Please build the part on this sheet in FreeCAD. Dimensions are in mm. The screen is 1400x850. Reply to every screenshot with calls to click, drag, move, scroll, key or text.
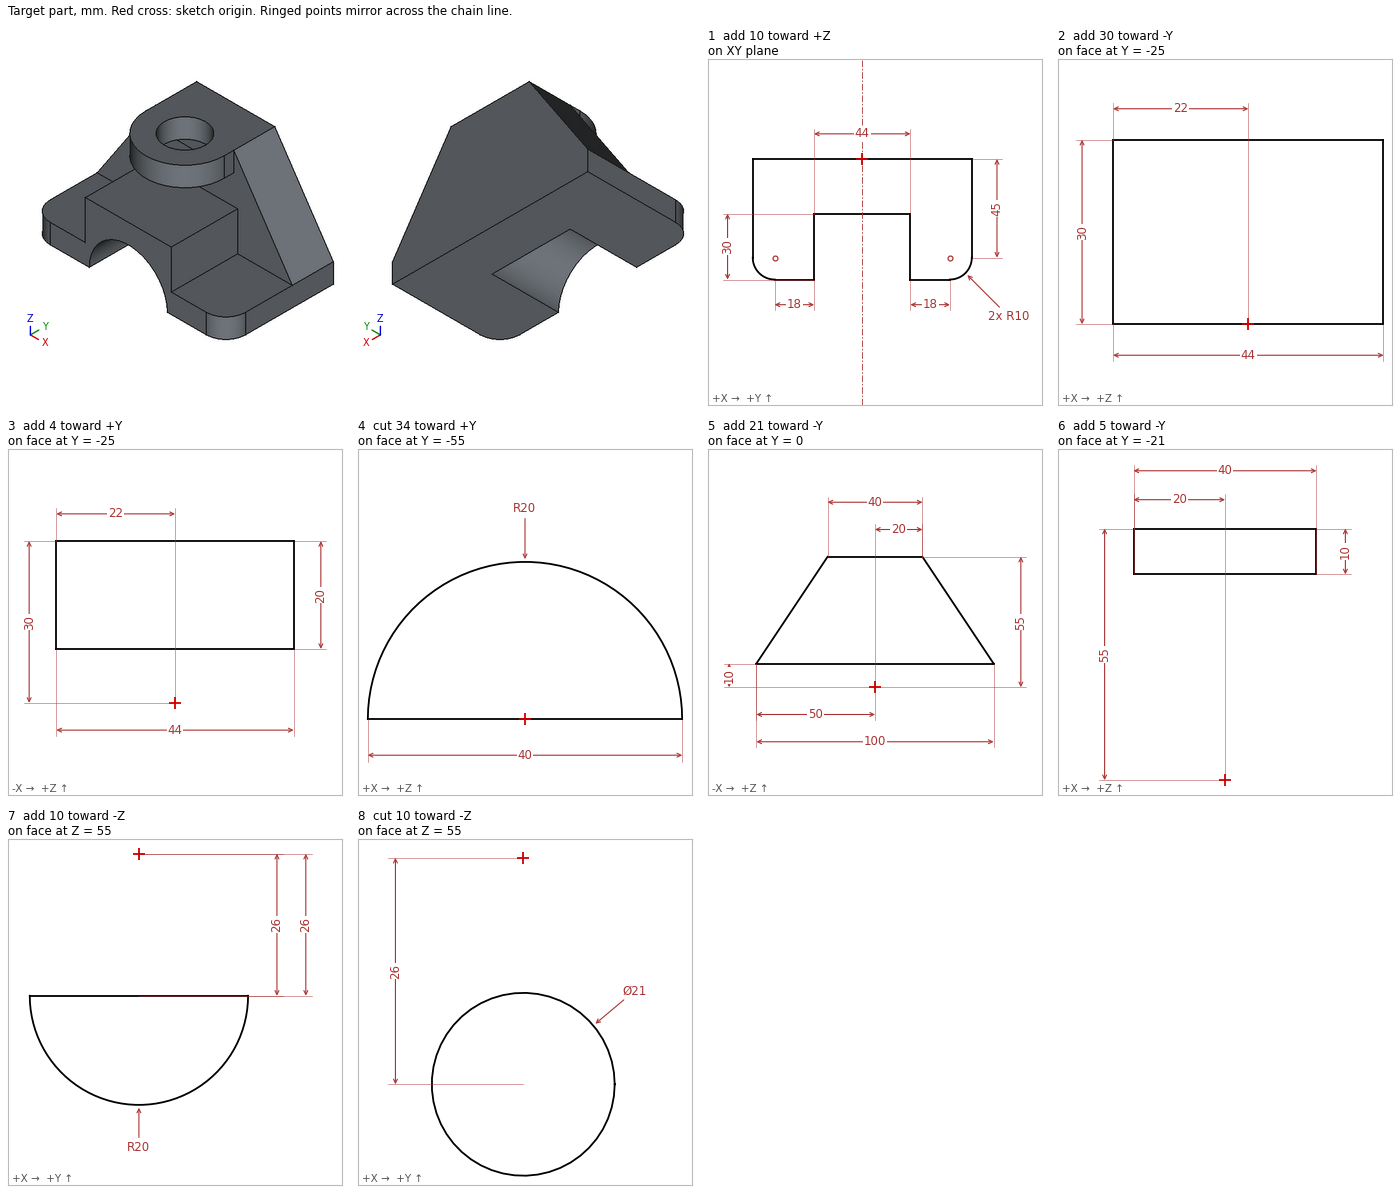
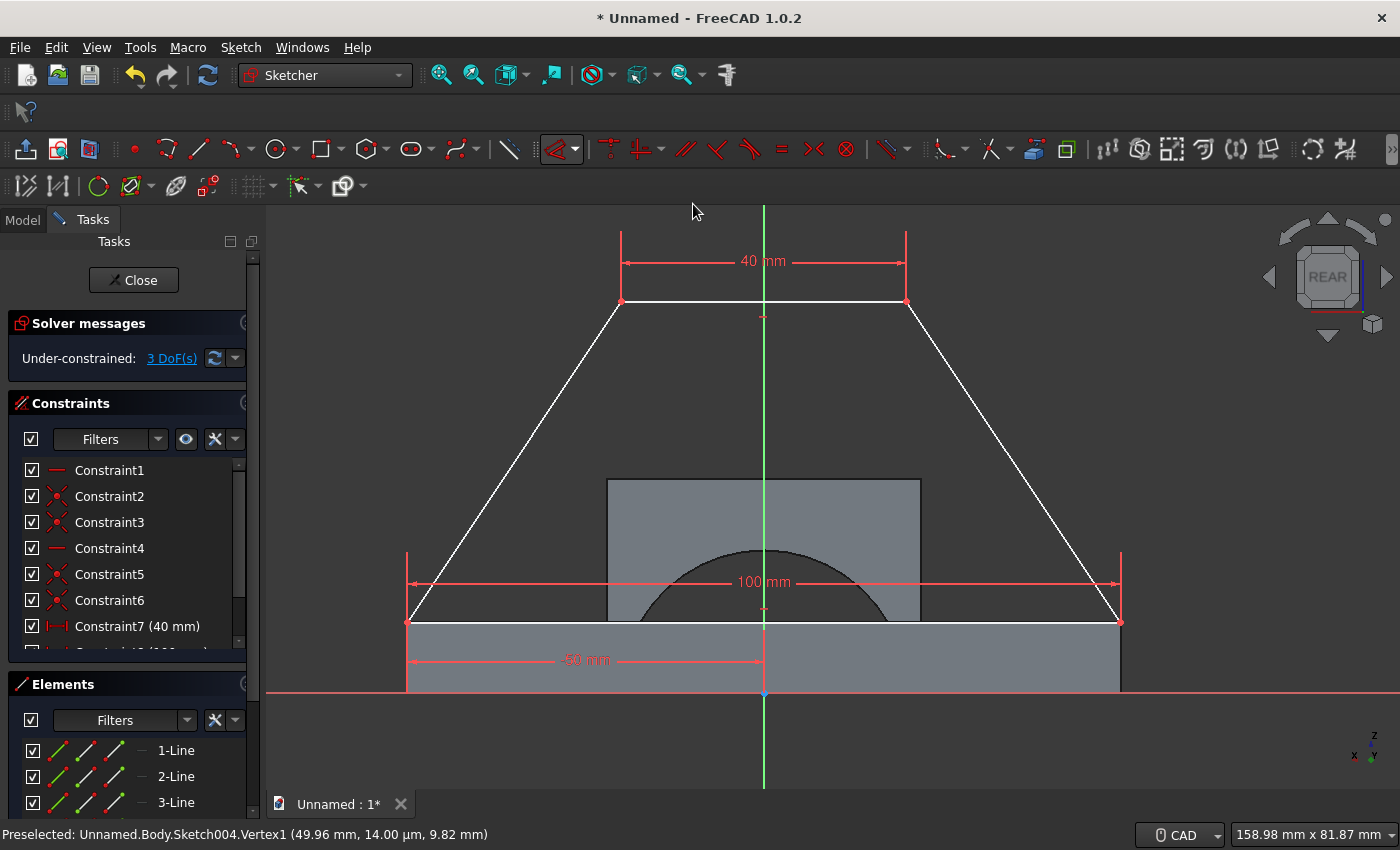
click(407, 623)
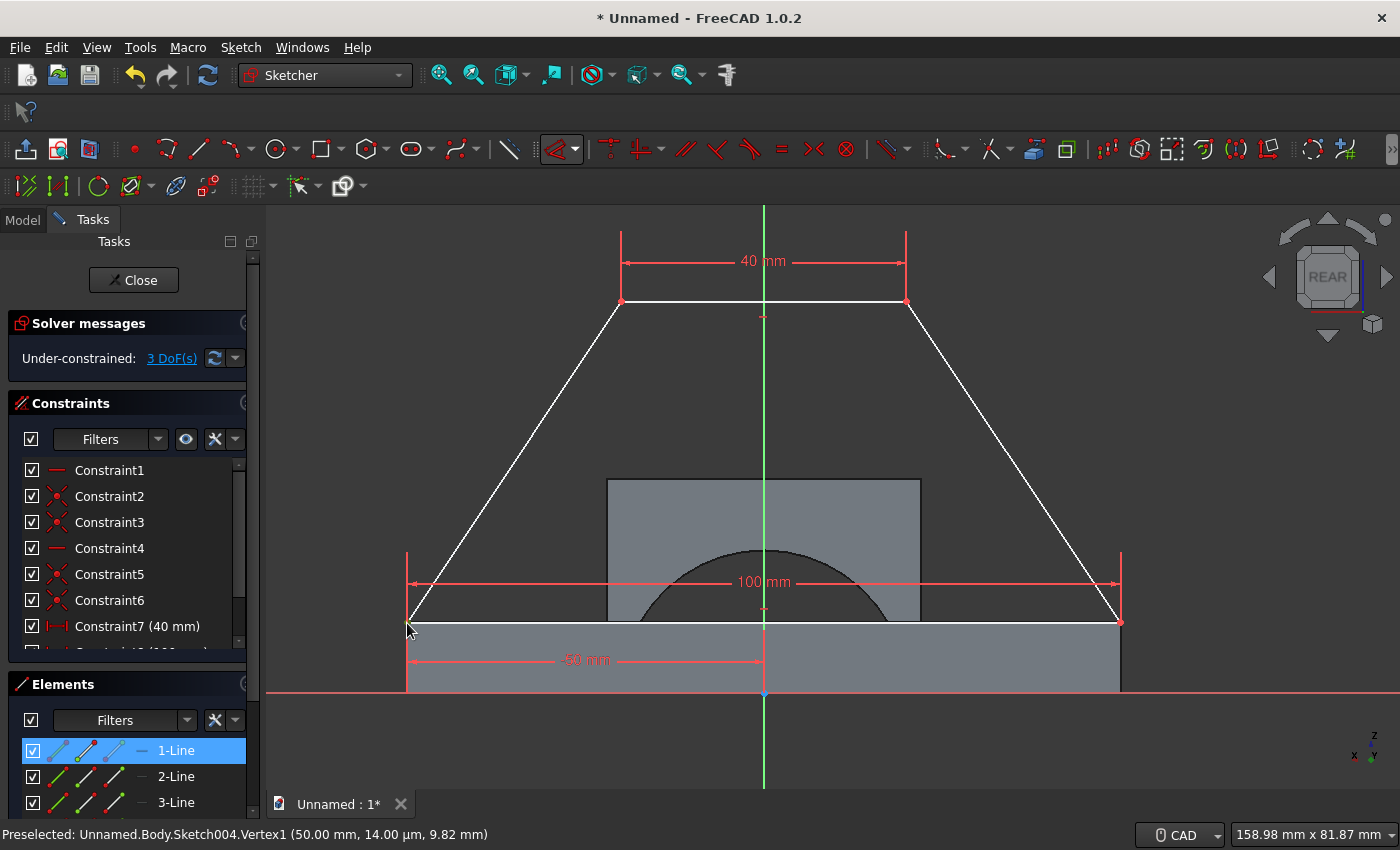
click(578, 150)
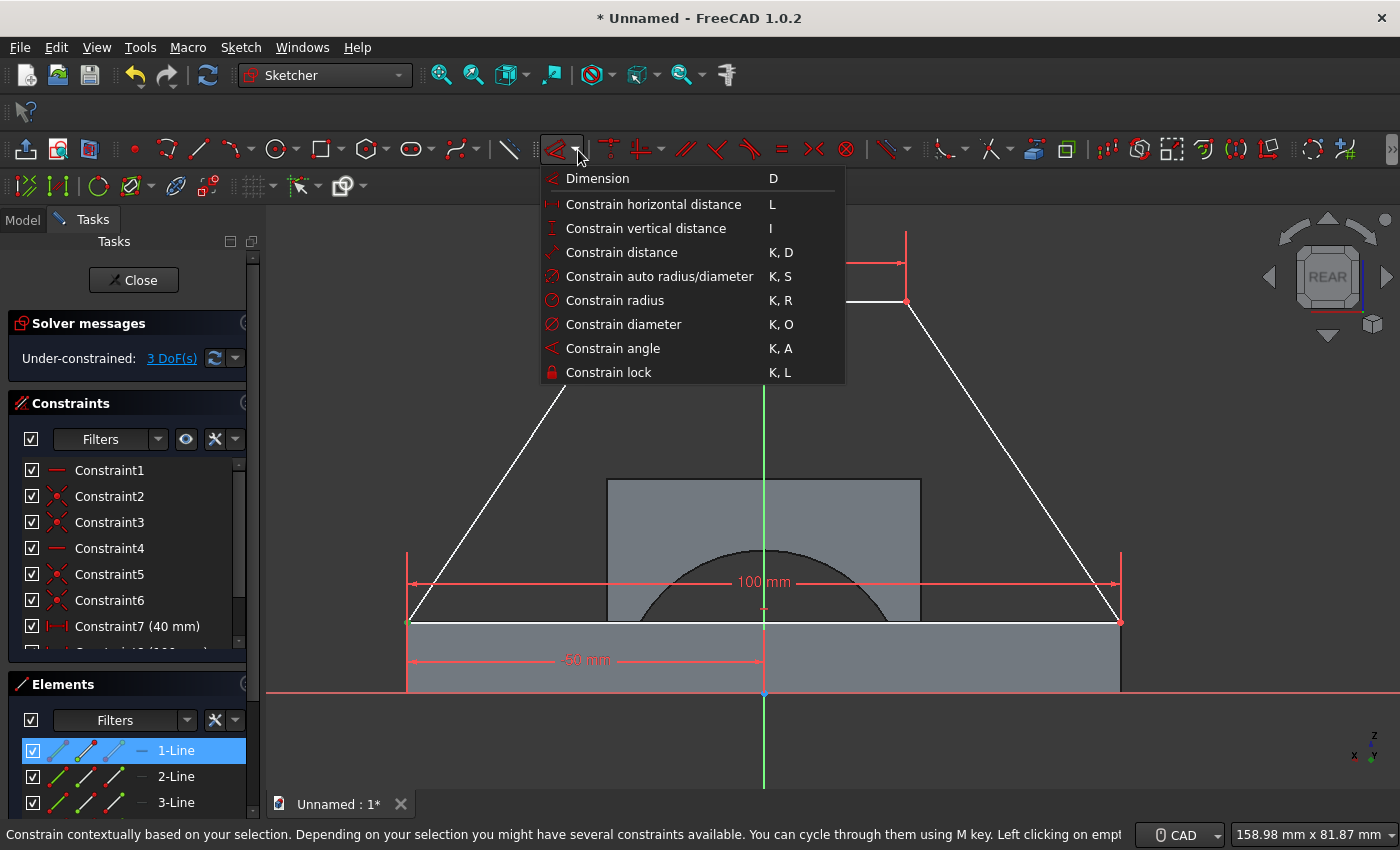
click(693, 228)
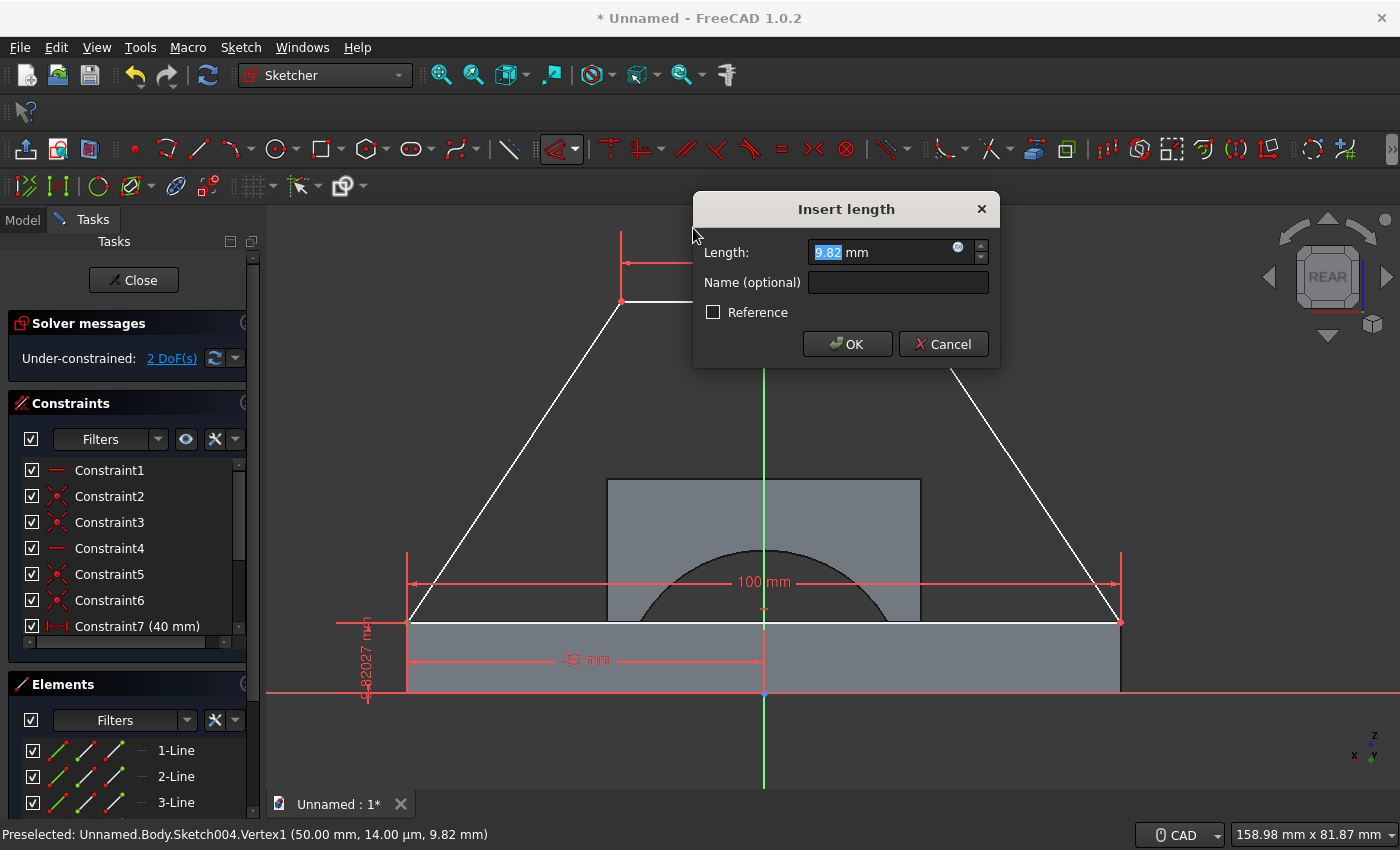
text(10)
key(Return)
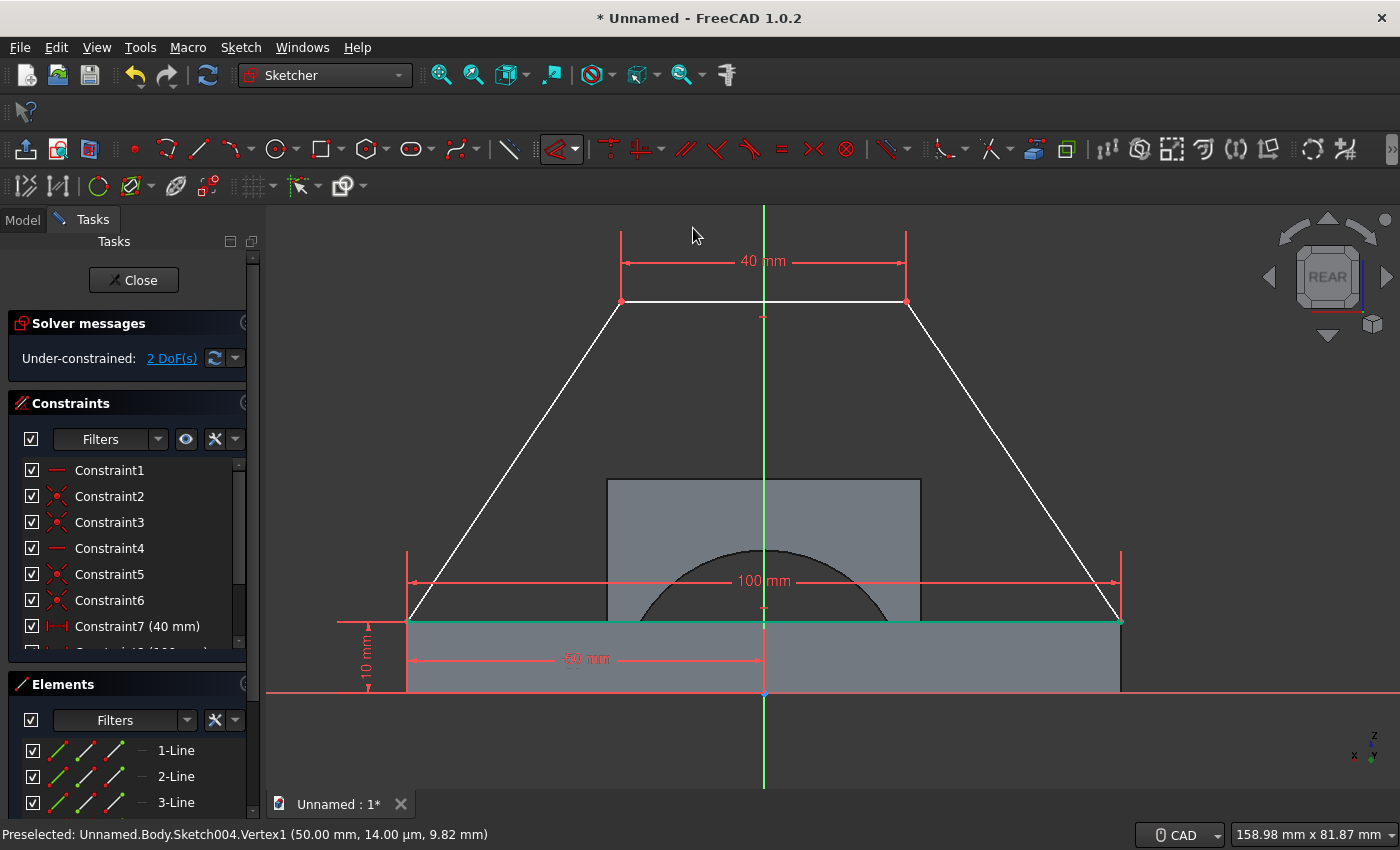
click(906, 302)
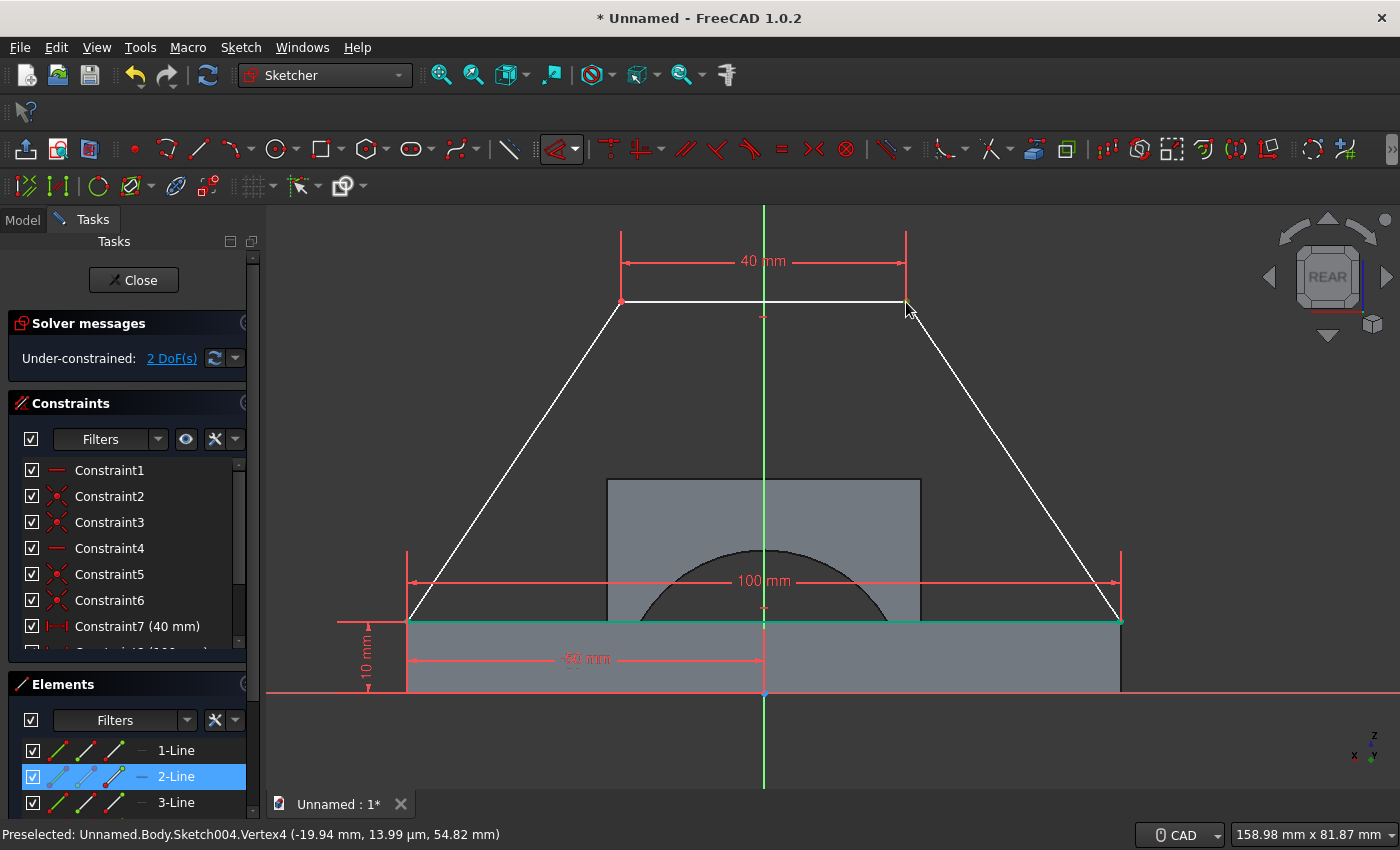
key(l)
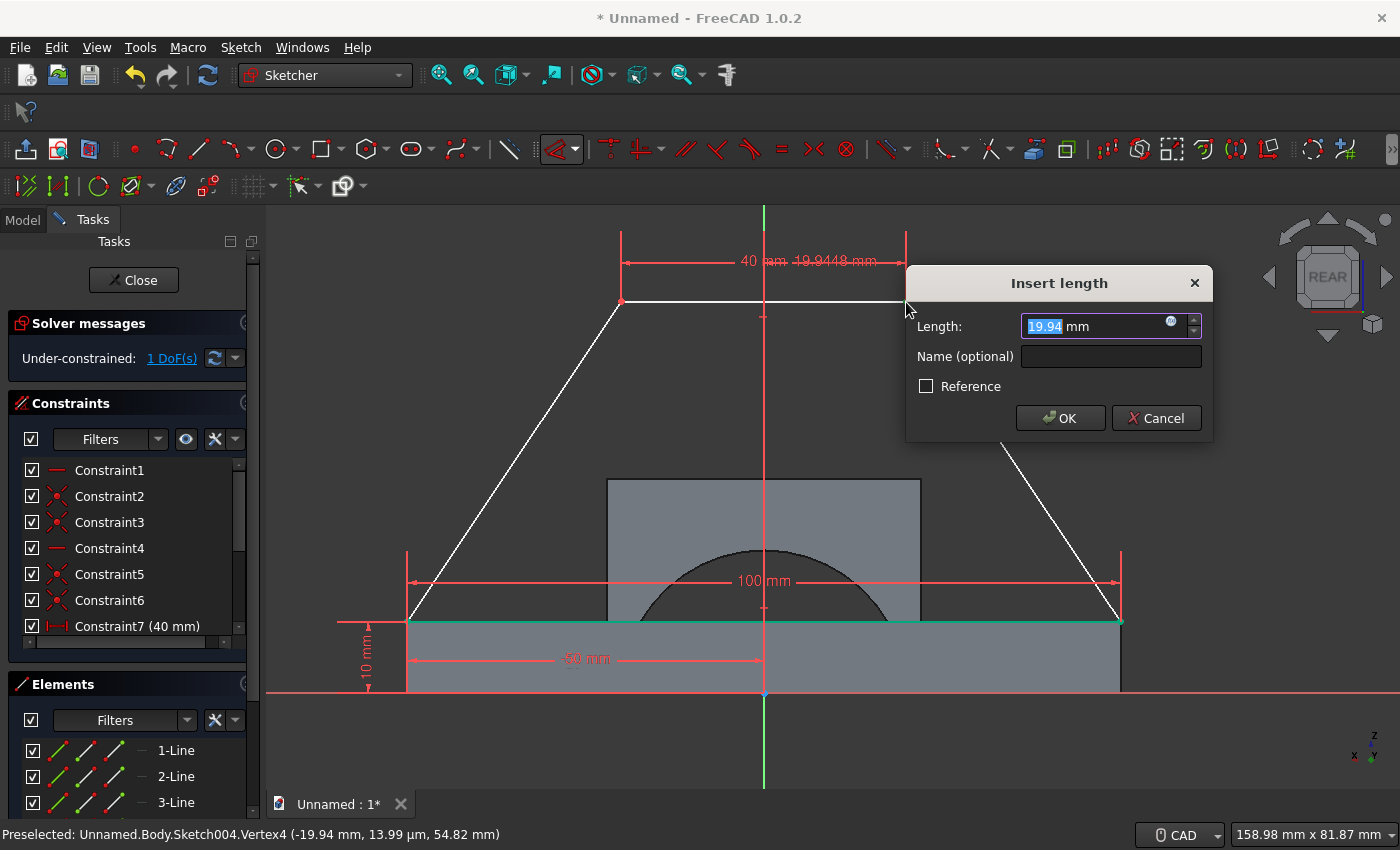
text(20)
key(Return)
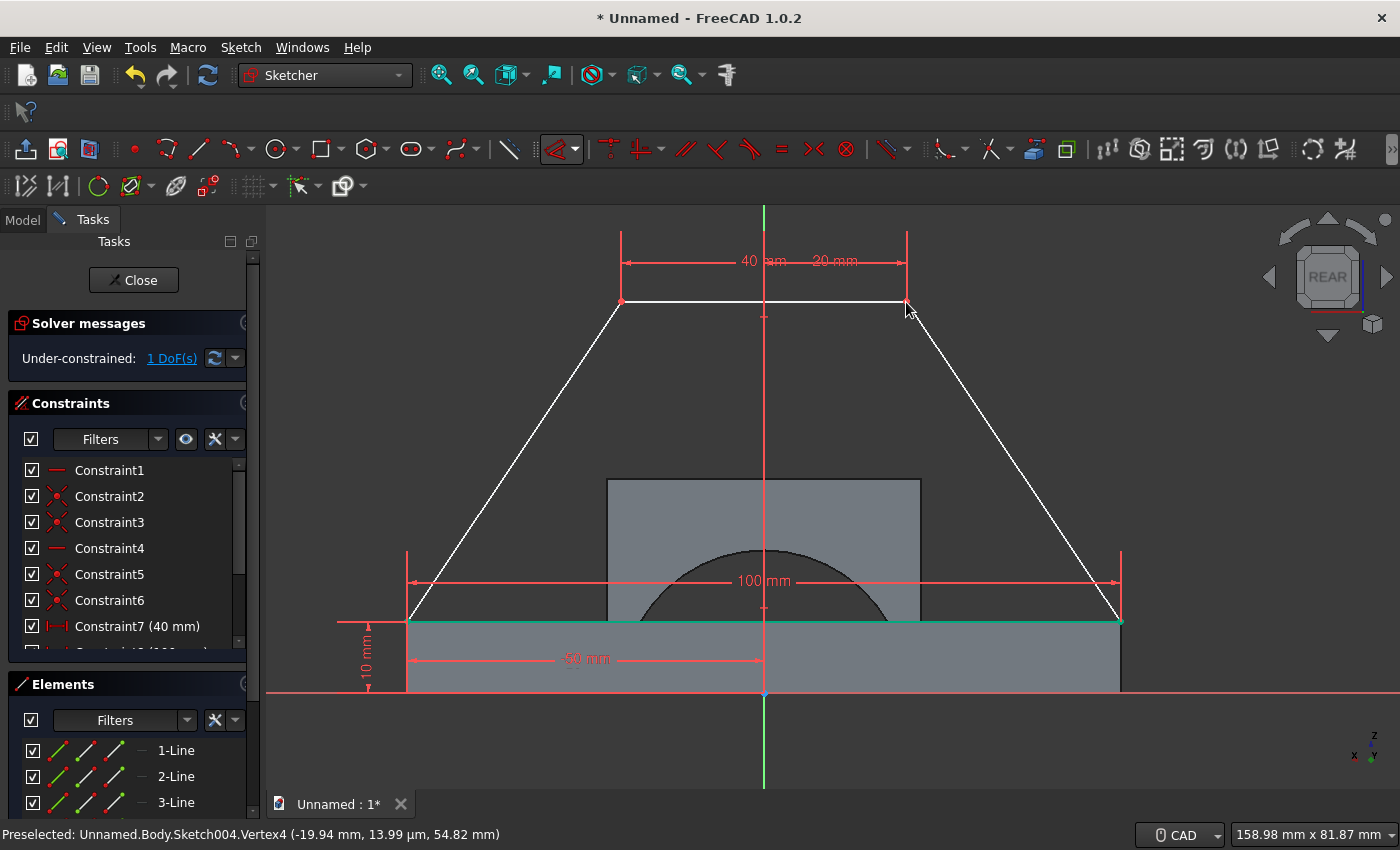
click(907, 302)